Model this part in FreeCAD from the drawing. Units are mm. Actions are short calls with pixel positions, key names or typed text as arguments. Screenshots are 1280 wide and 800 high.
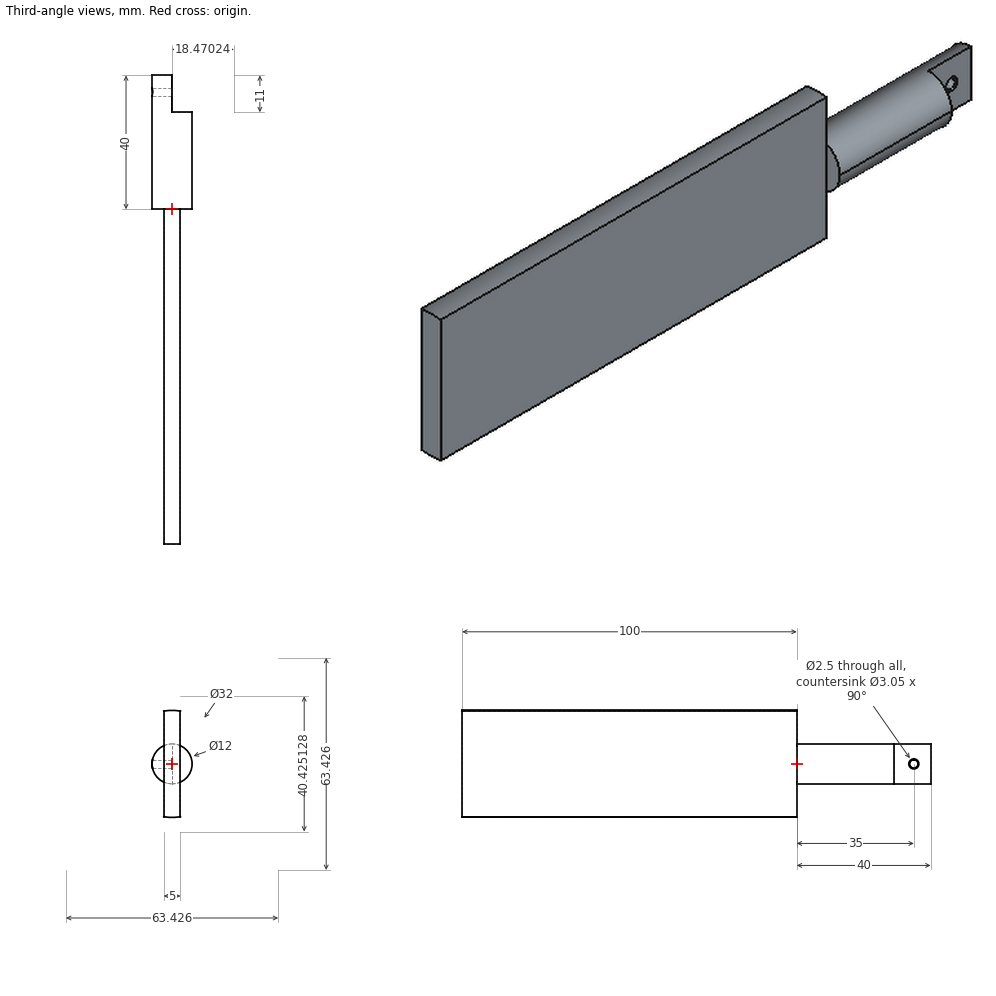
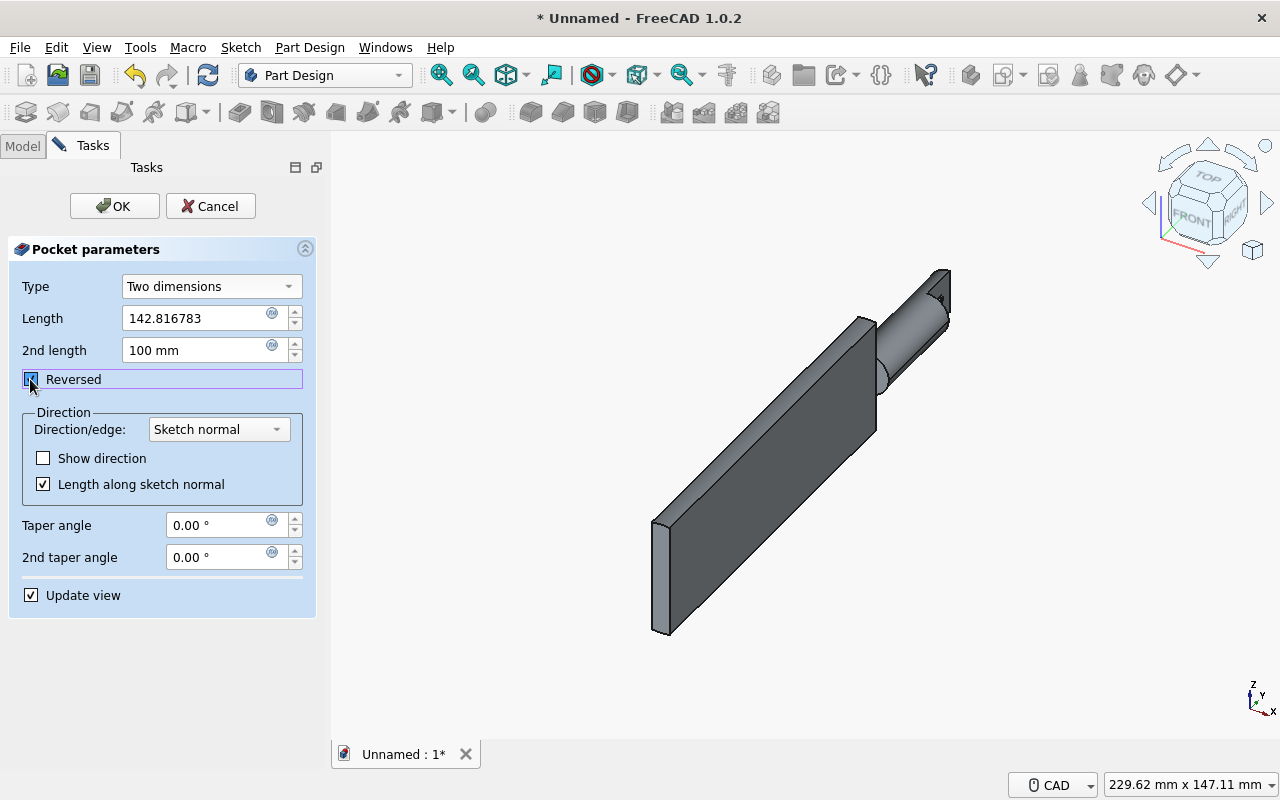
click(115, 206)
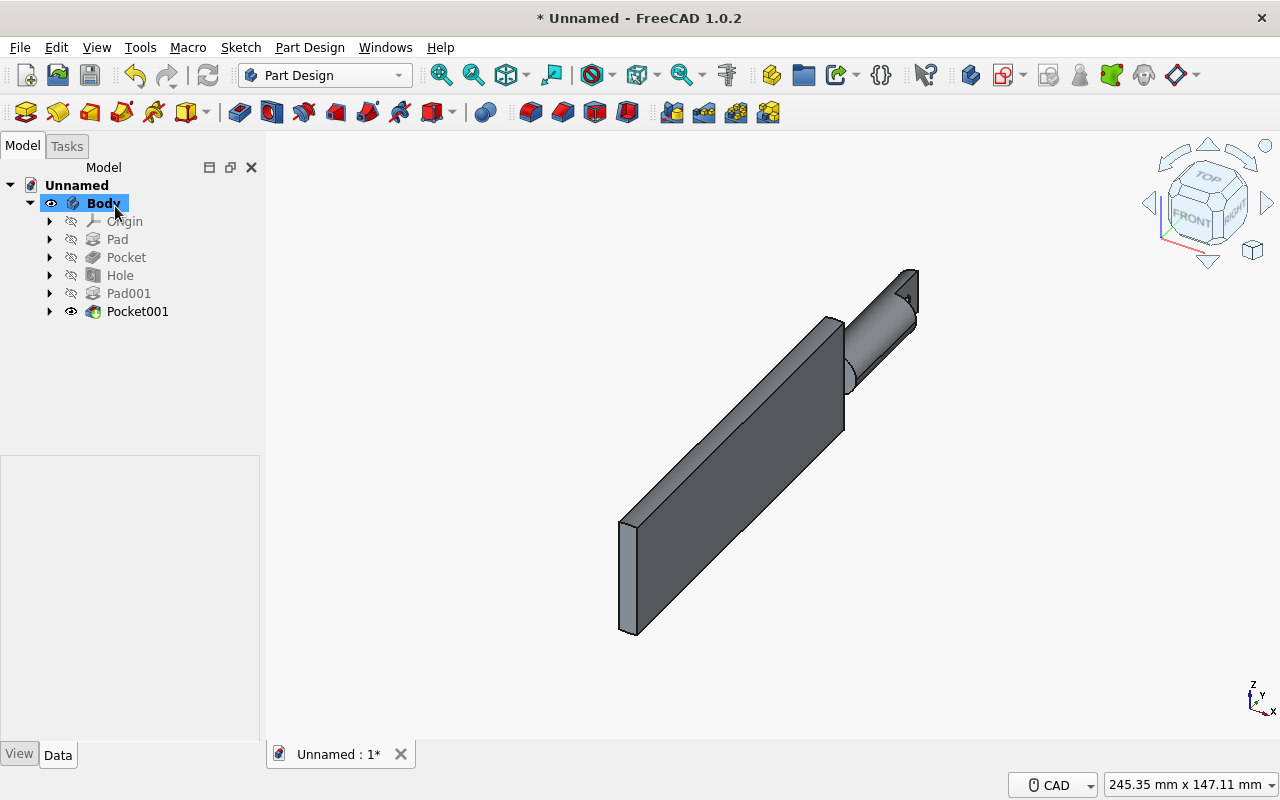
key(0)